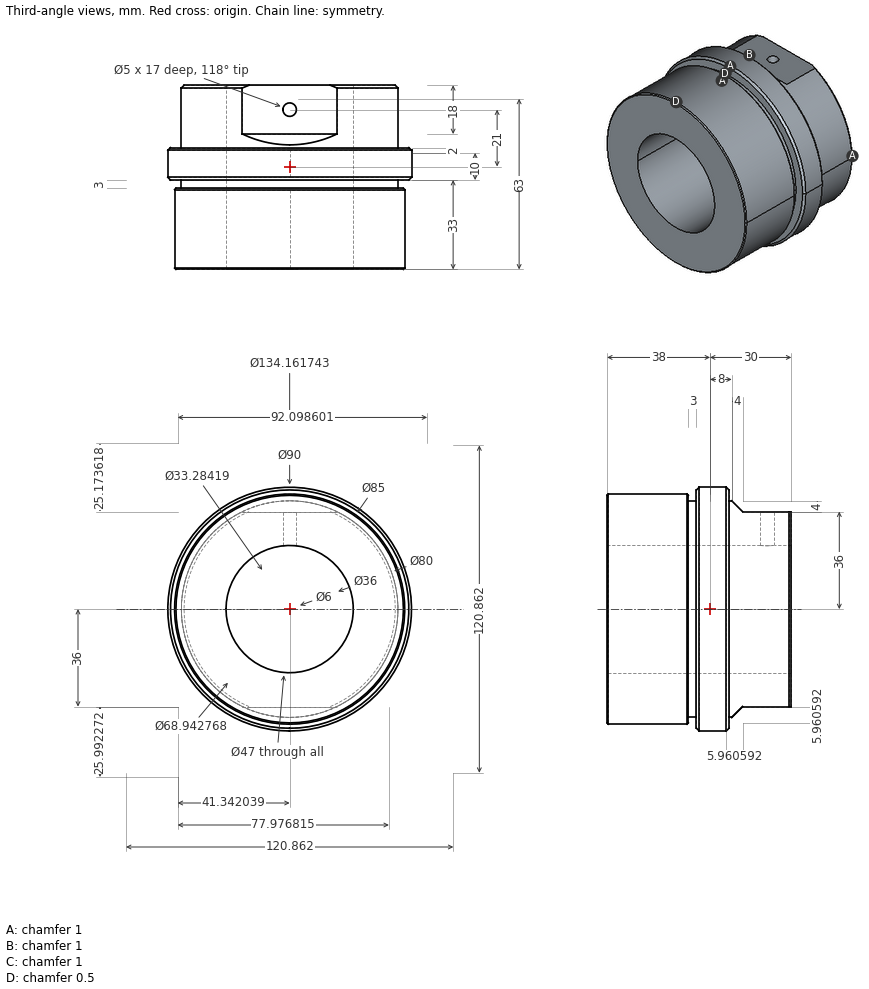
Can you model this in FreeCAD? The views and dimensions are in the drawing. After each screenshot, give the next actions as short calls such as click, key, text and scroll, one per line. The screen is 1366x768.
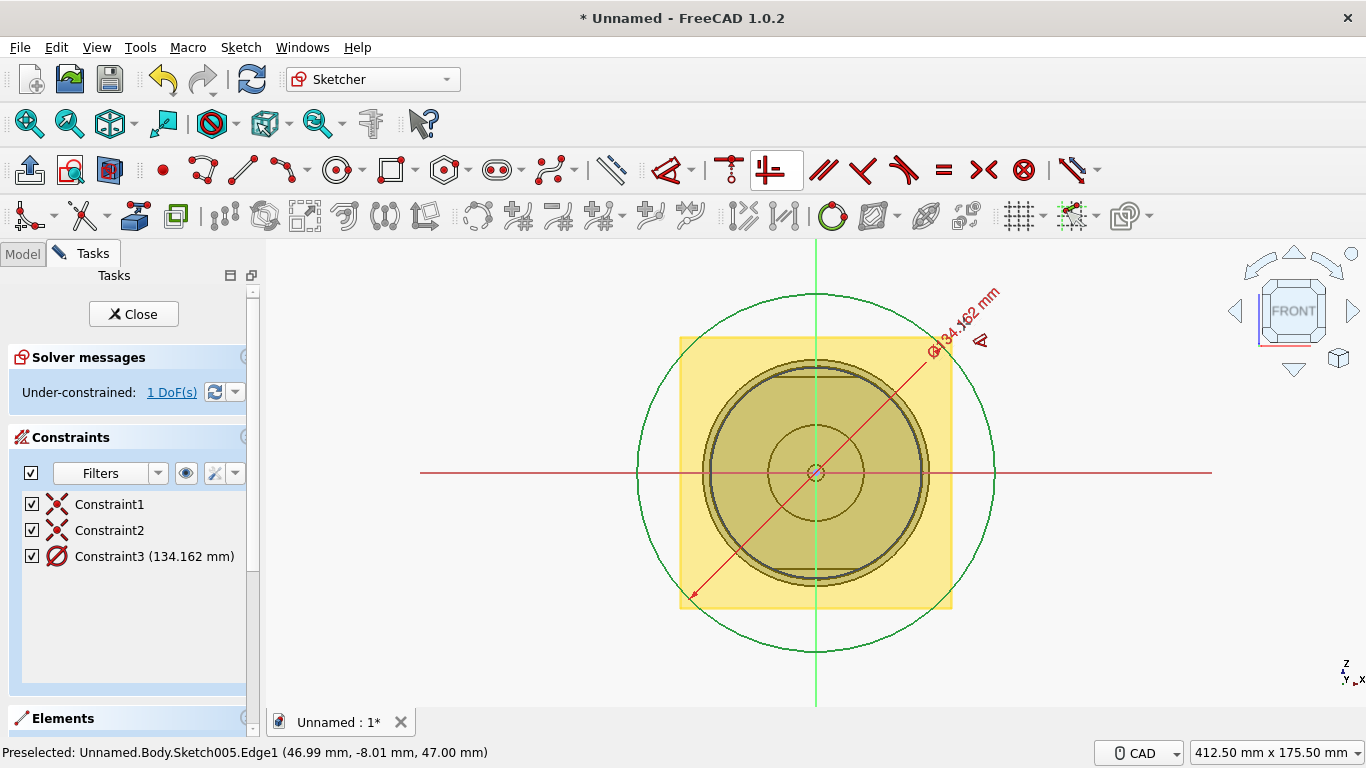
click(890, 398)
click(912, 375)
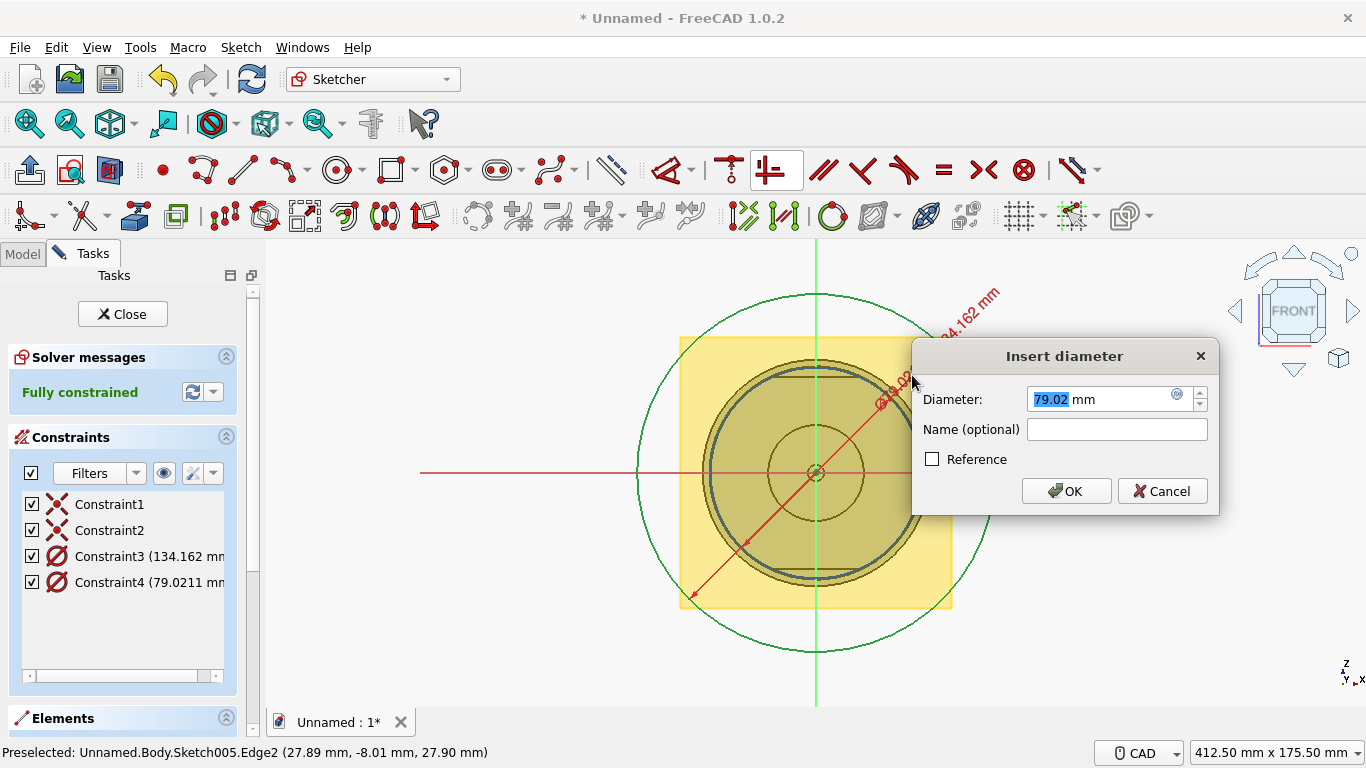
text(80)
key(Return)
key(Escape)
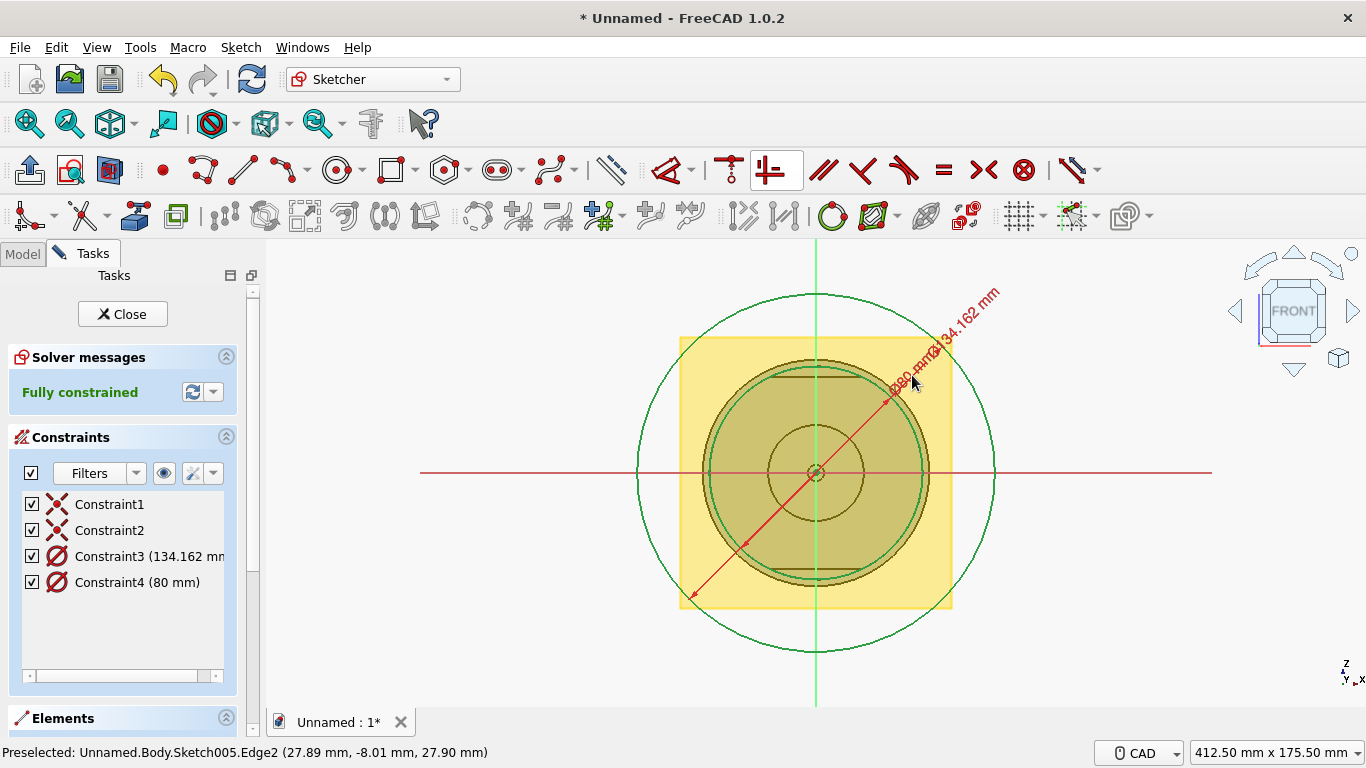
click(123, 314)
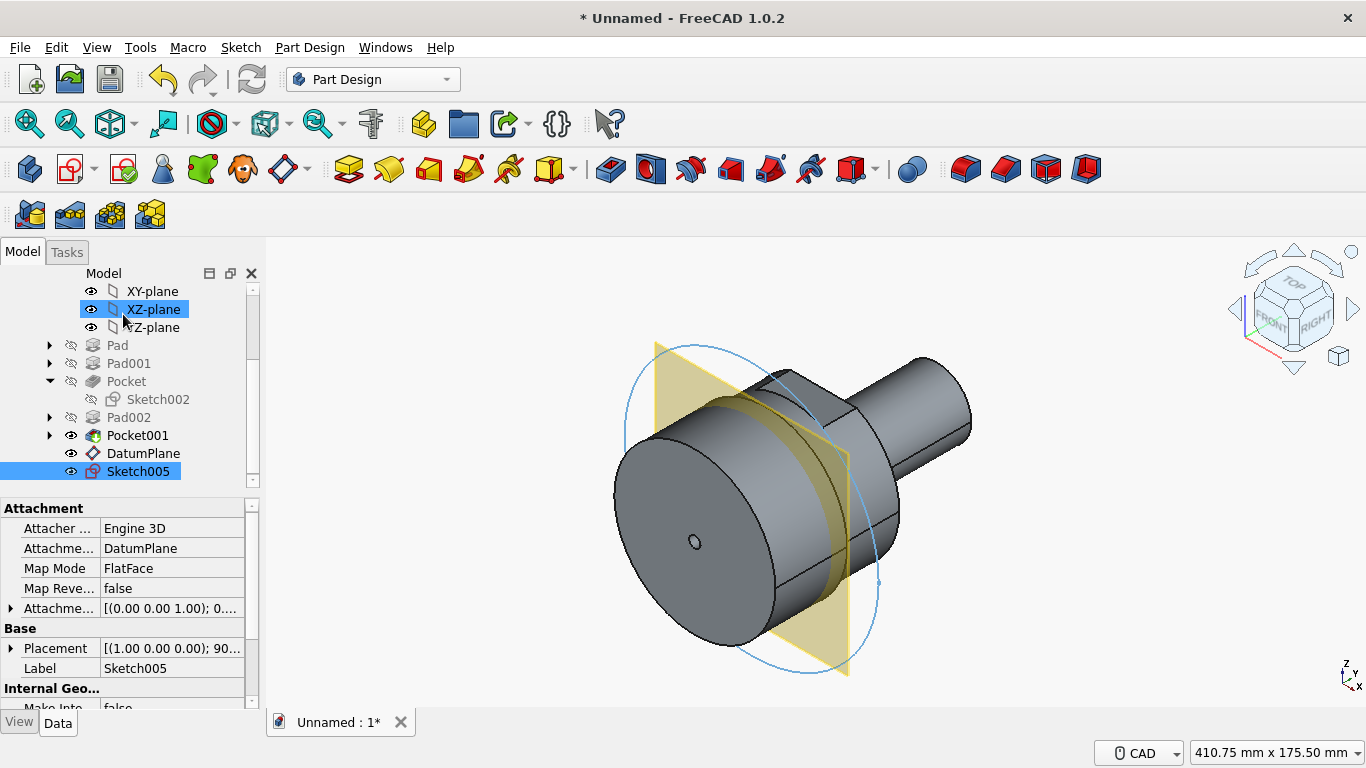
click(612, 170)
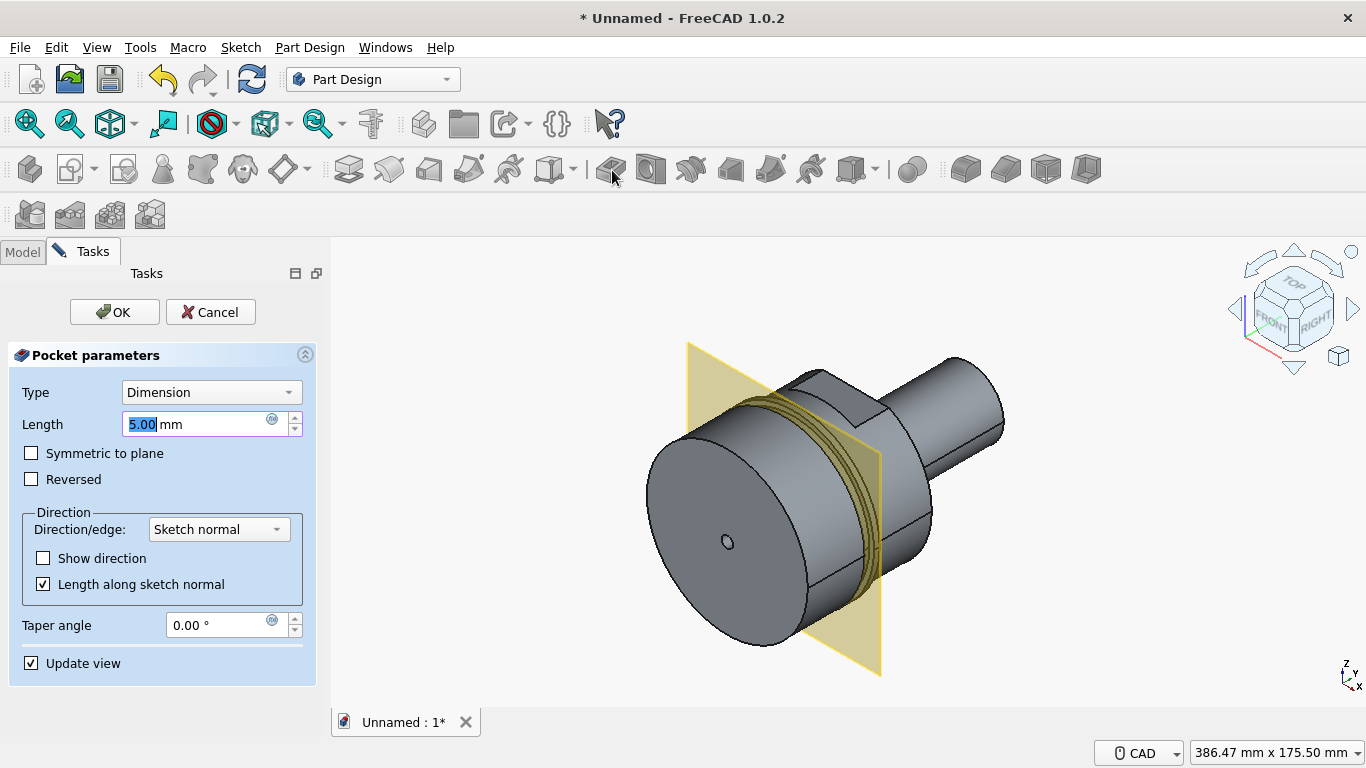
text(3)
key(Tab)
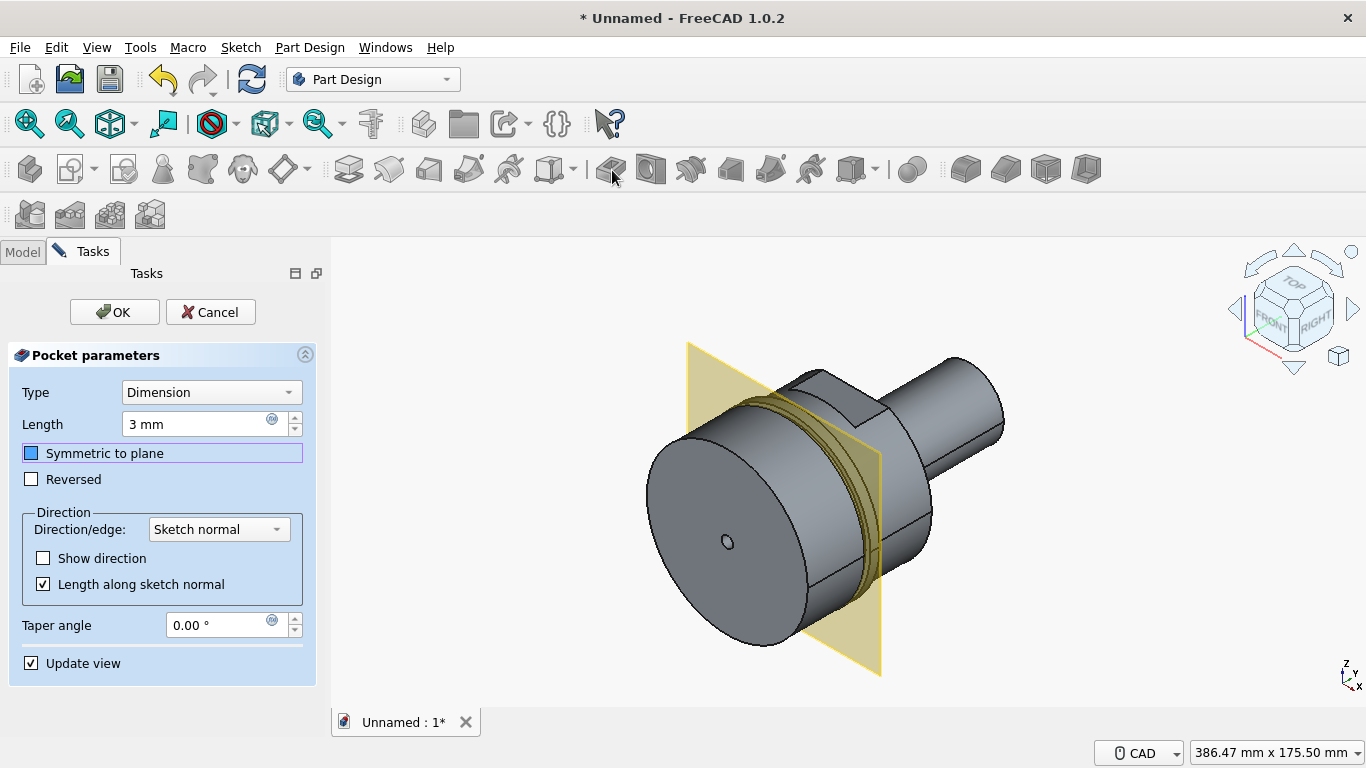
click(115, 312)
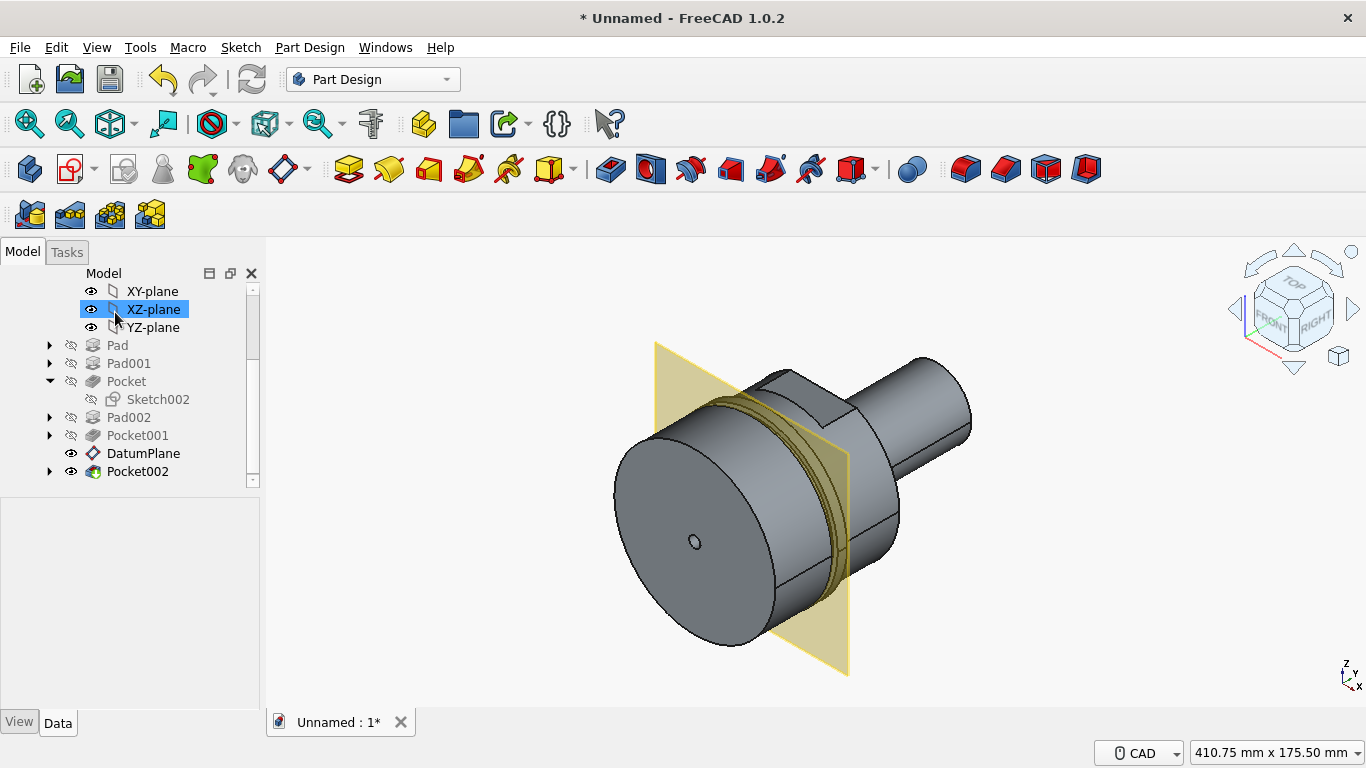
click(116, 453)
key(space)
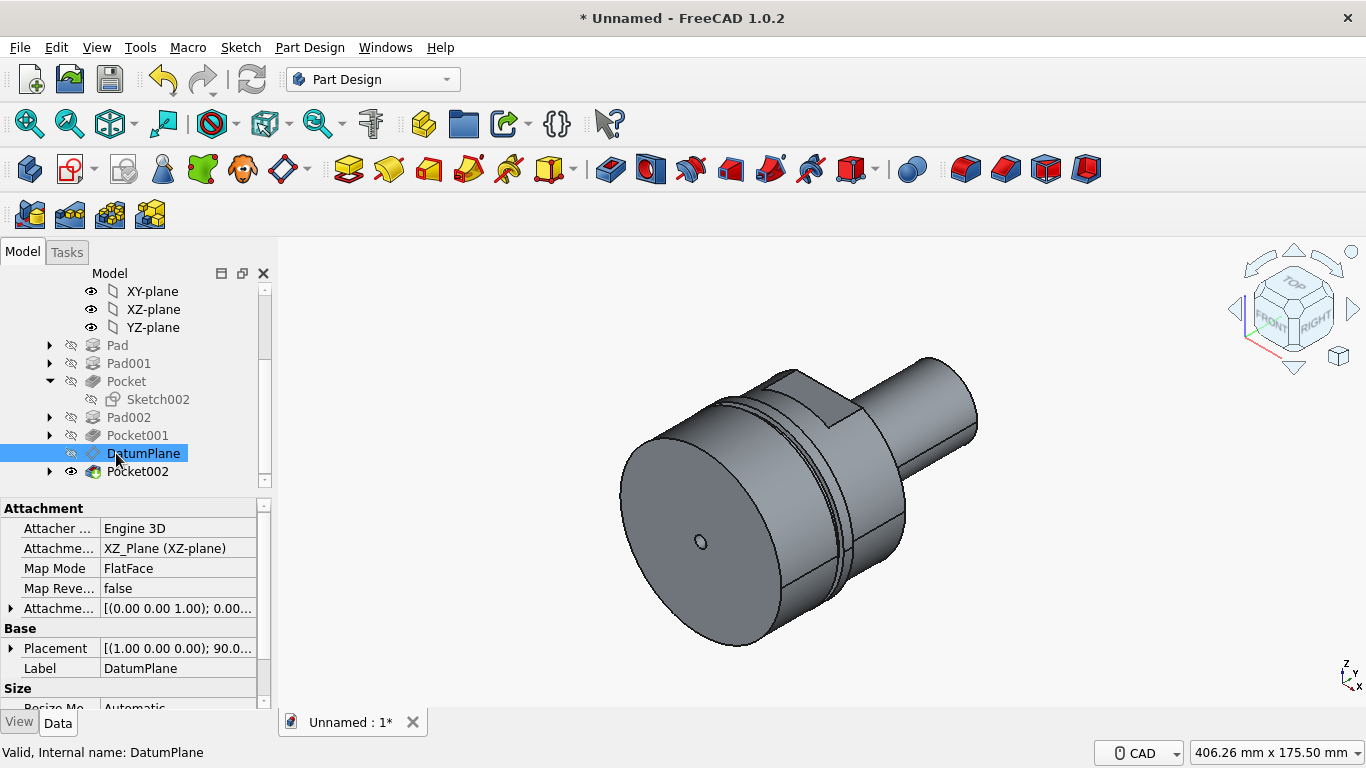
scroll(160, 377, down, 3)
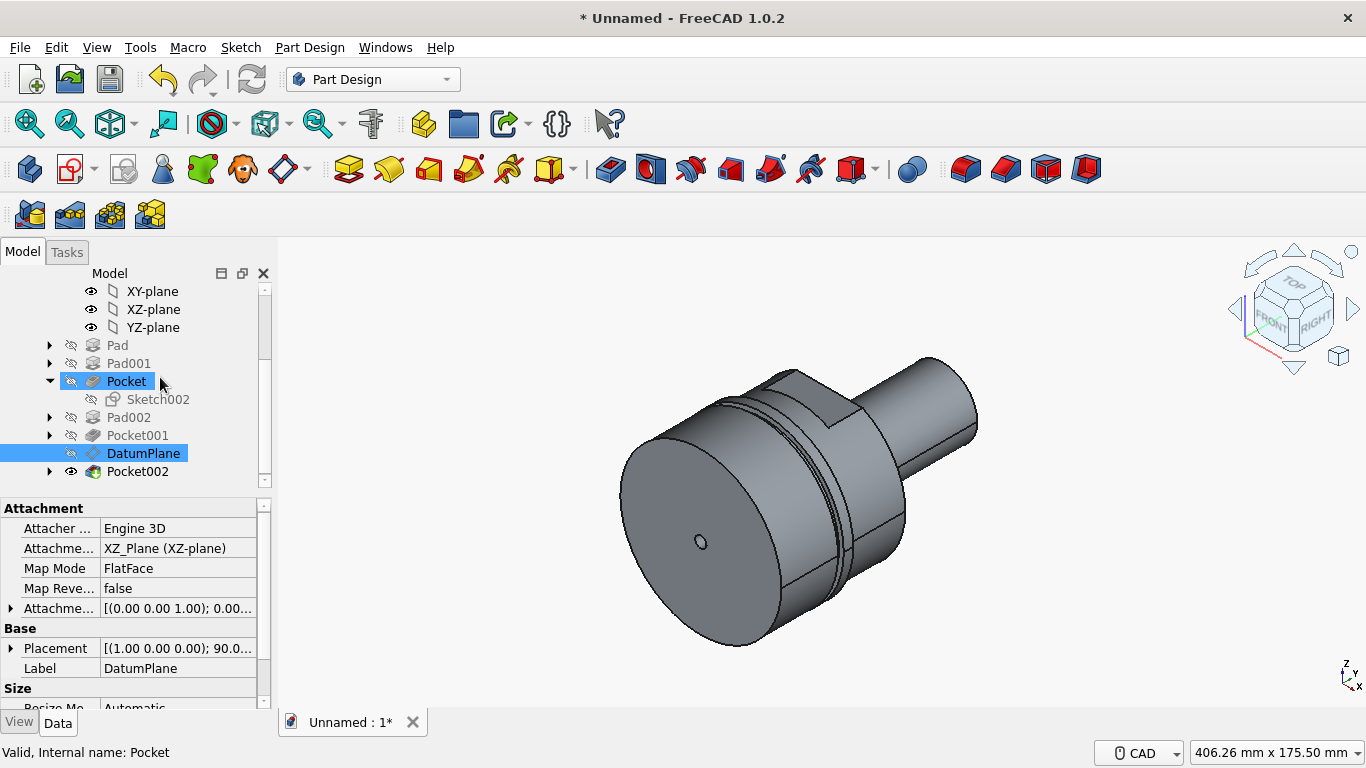
scroll(160, 377, up, 15)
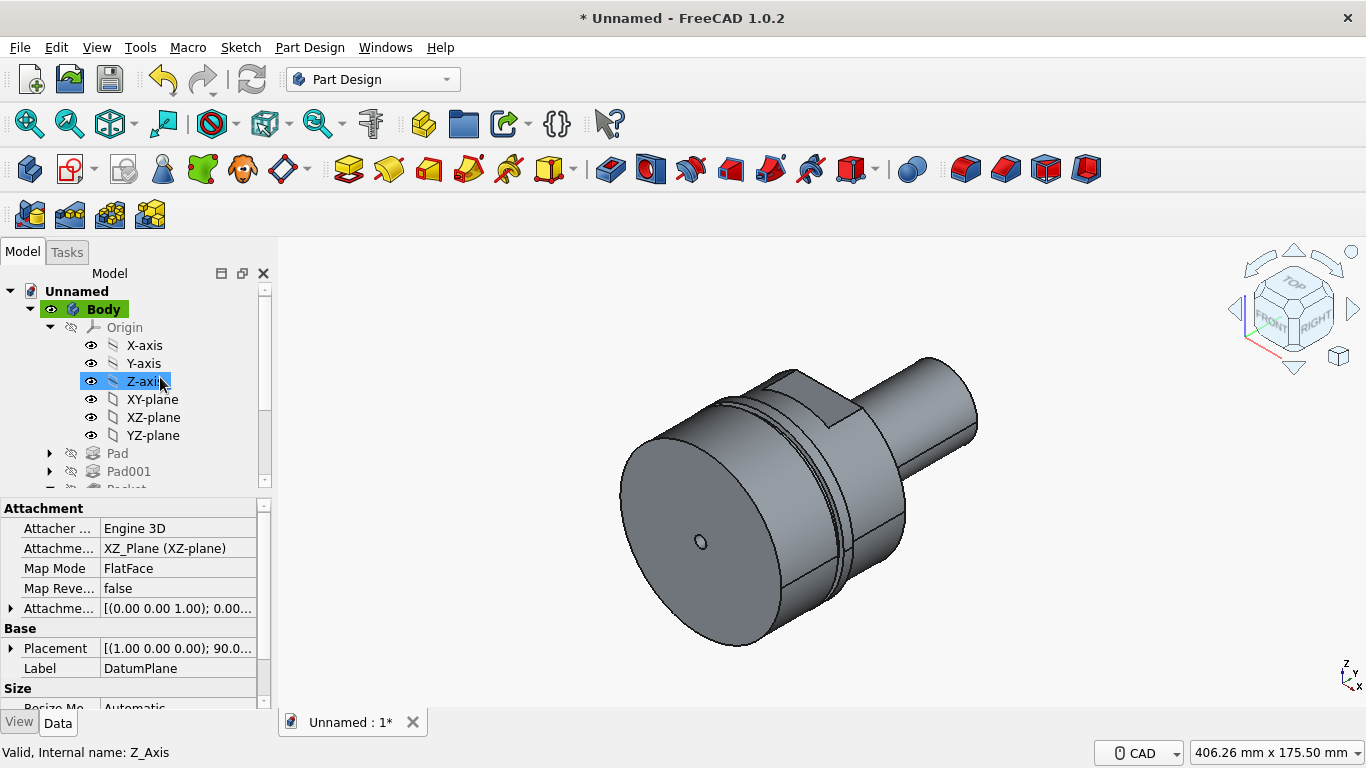
click(136, 417)